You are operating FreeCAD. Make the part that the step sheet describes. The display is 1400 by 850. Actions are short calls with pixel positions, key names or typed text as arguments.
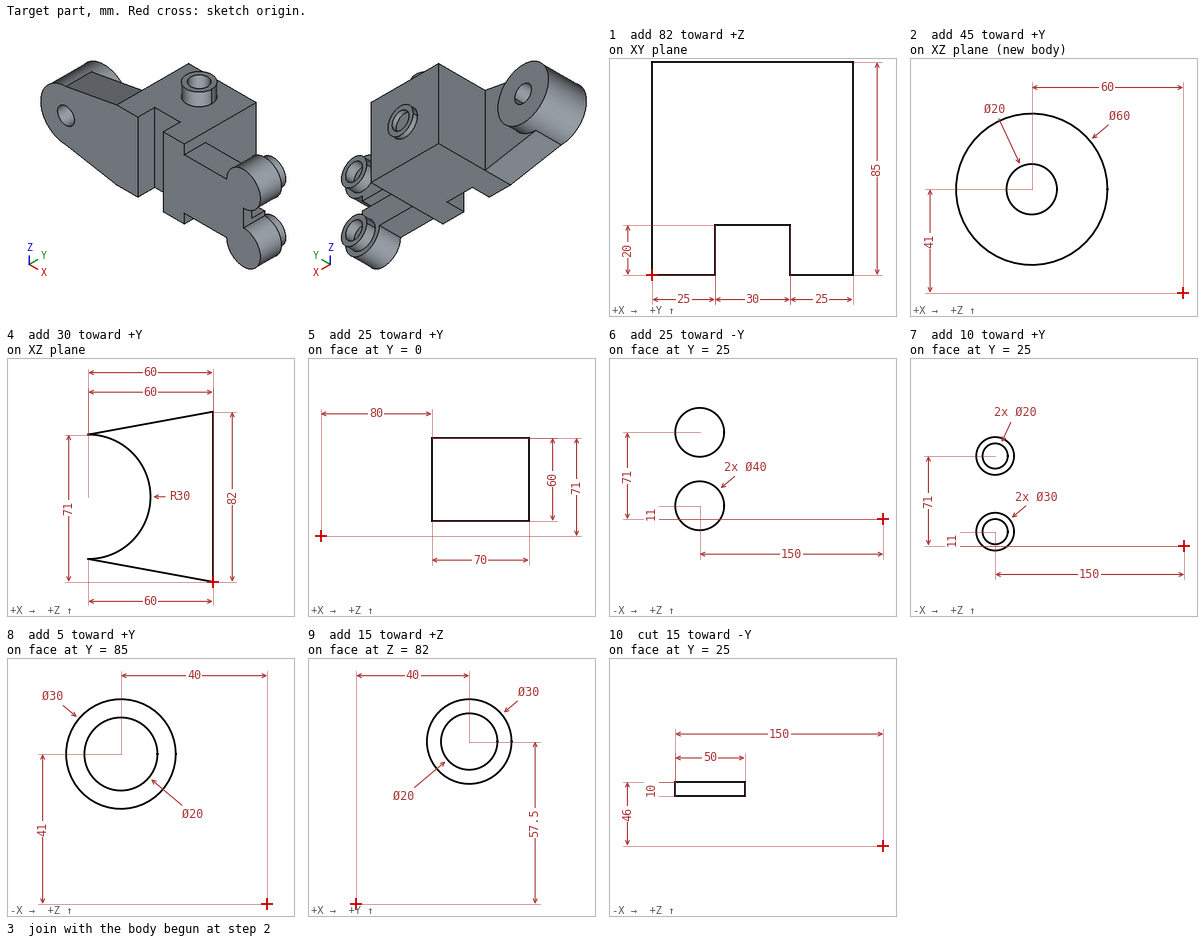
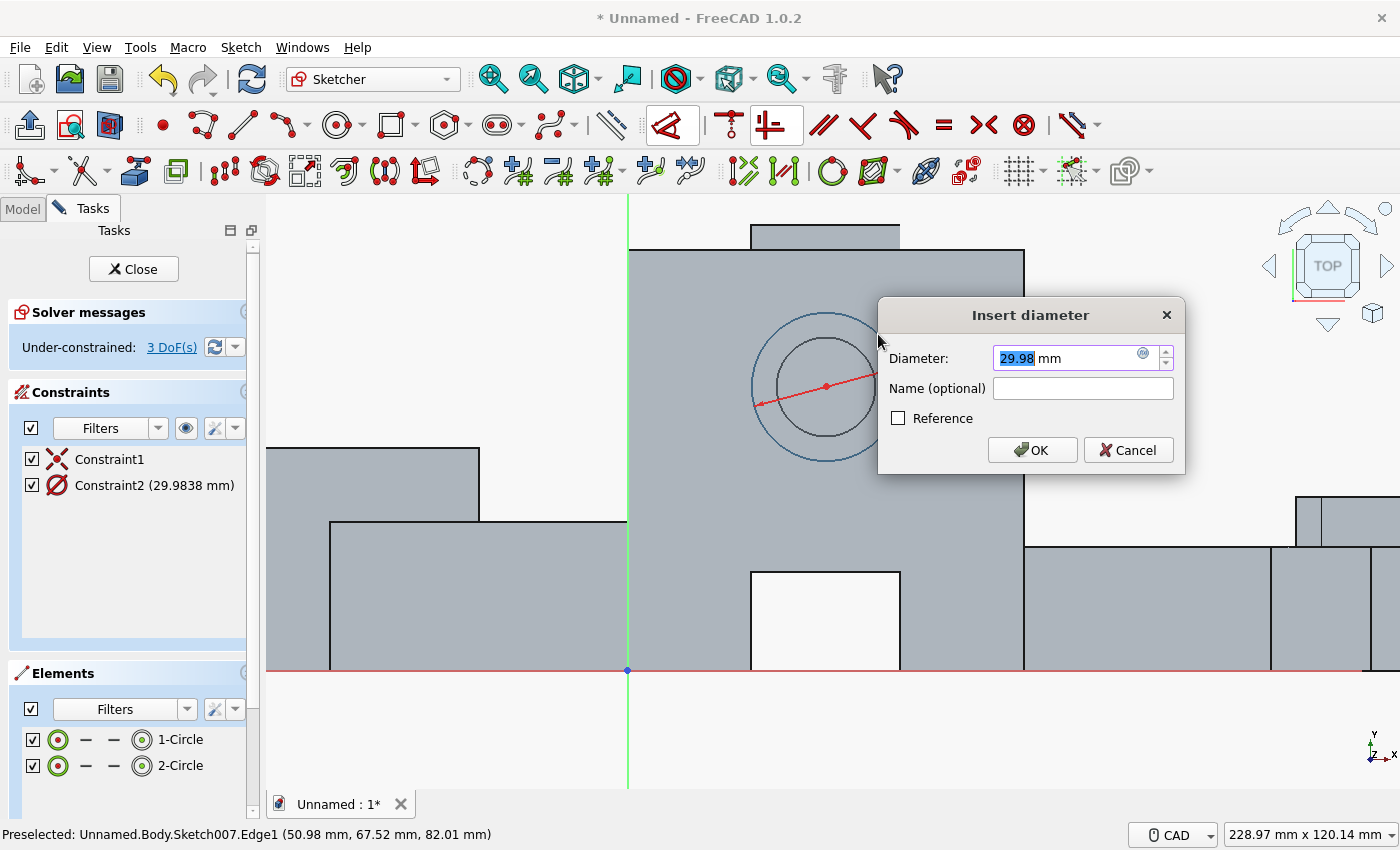
text(30)
key(Return)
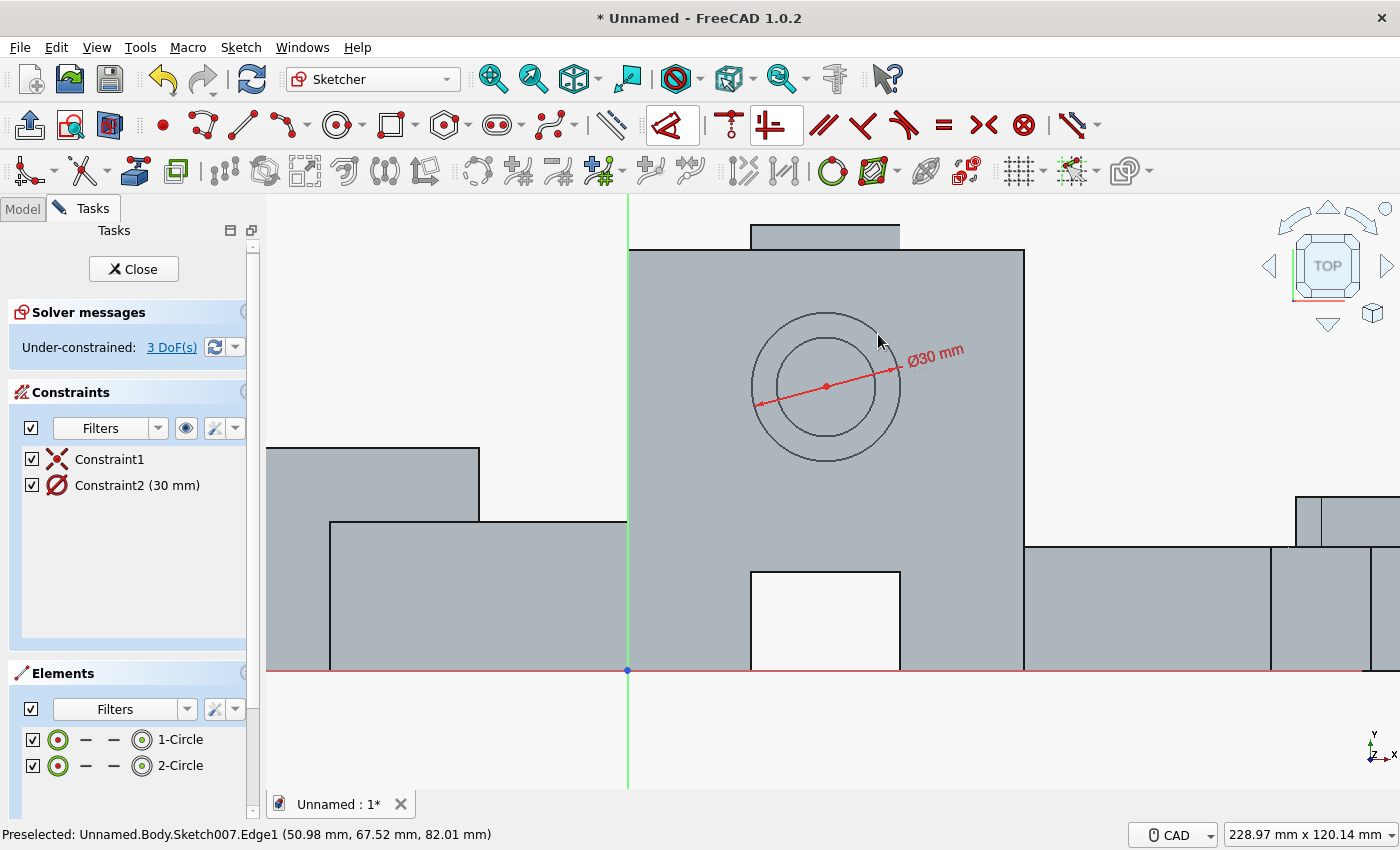
click(861, 352)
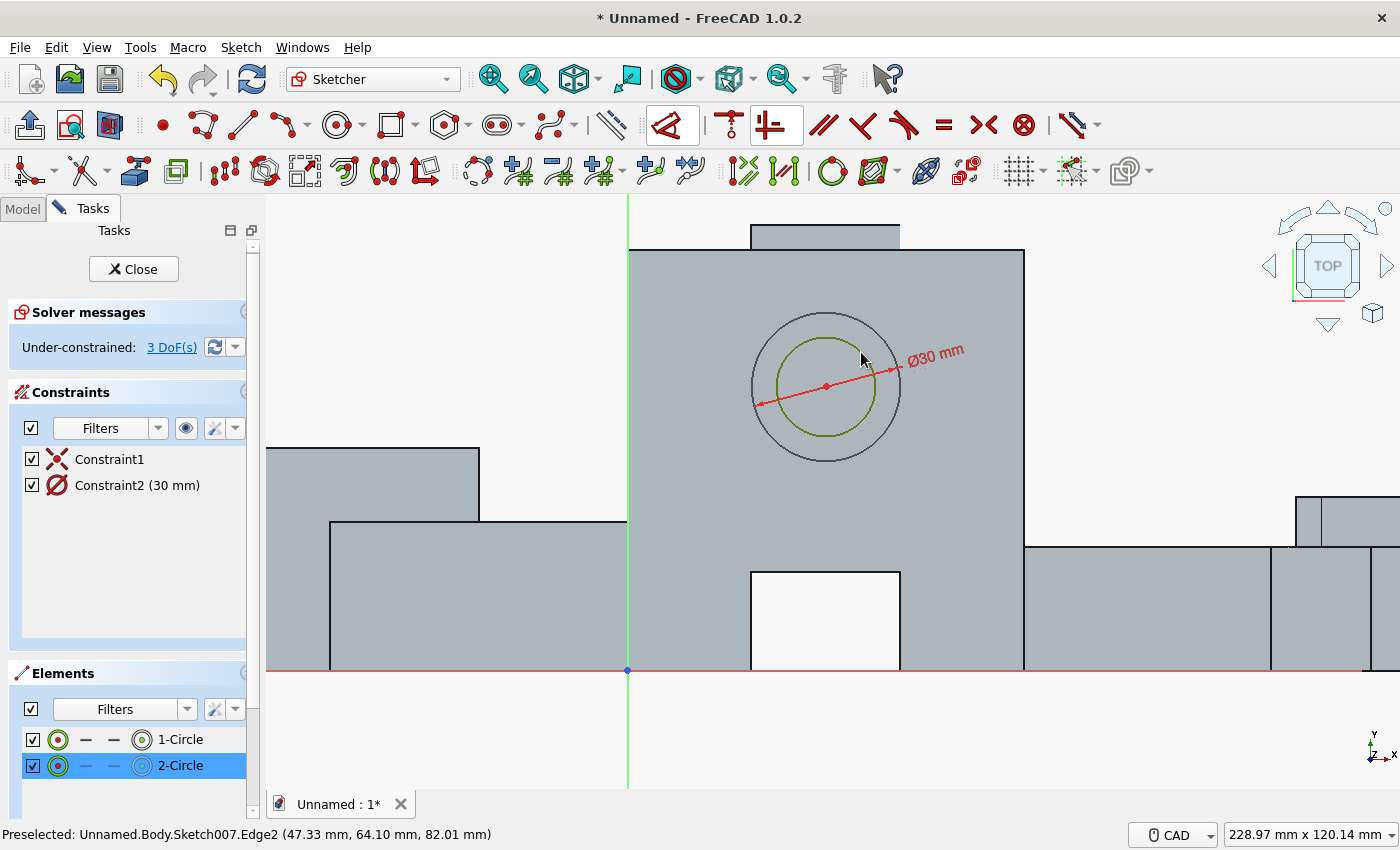
key(k)
key(o)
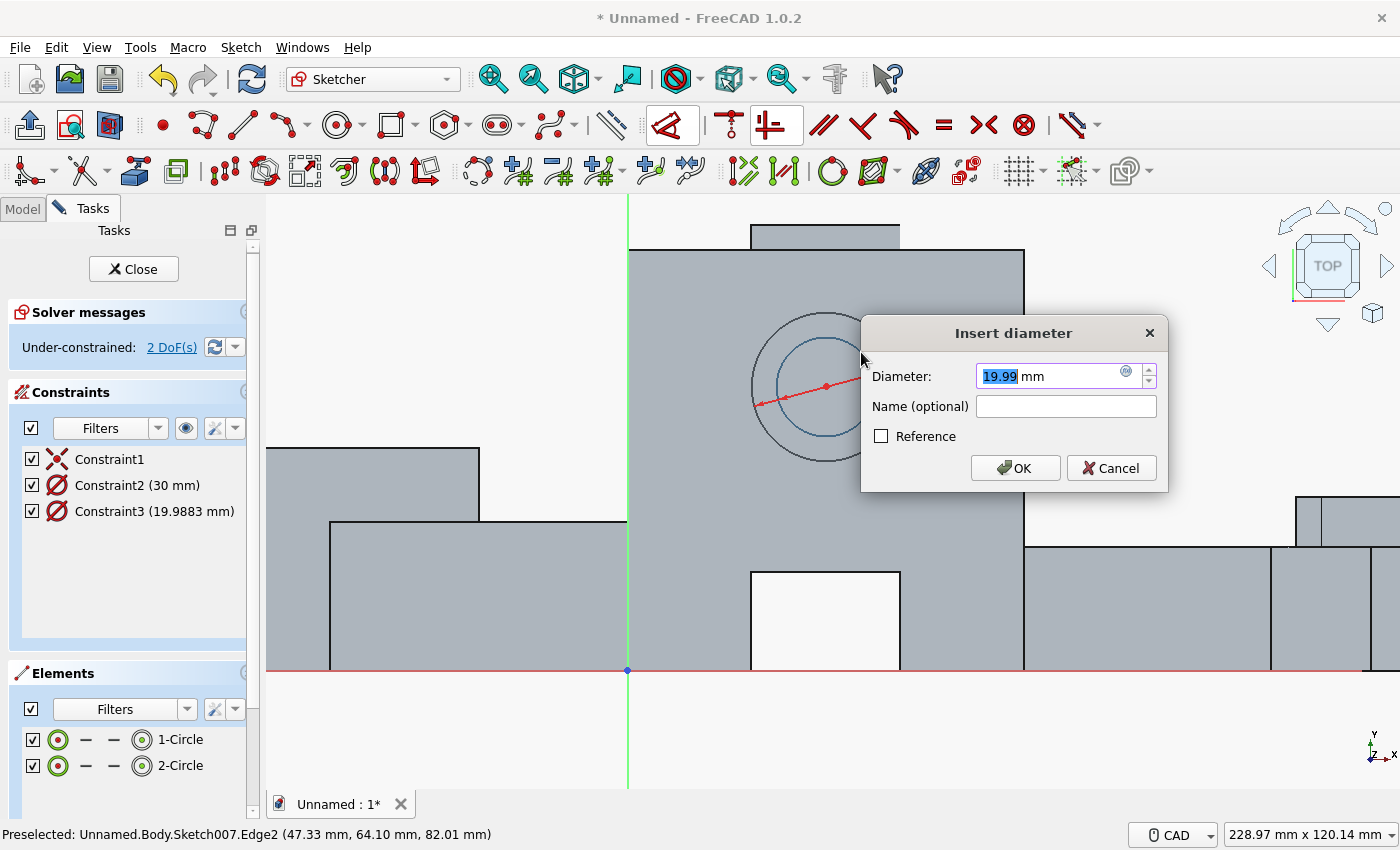
text(20)
key(Return)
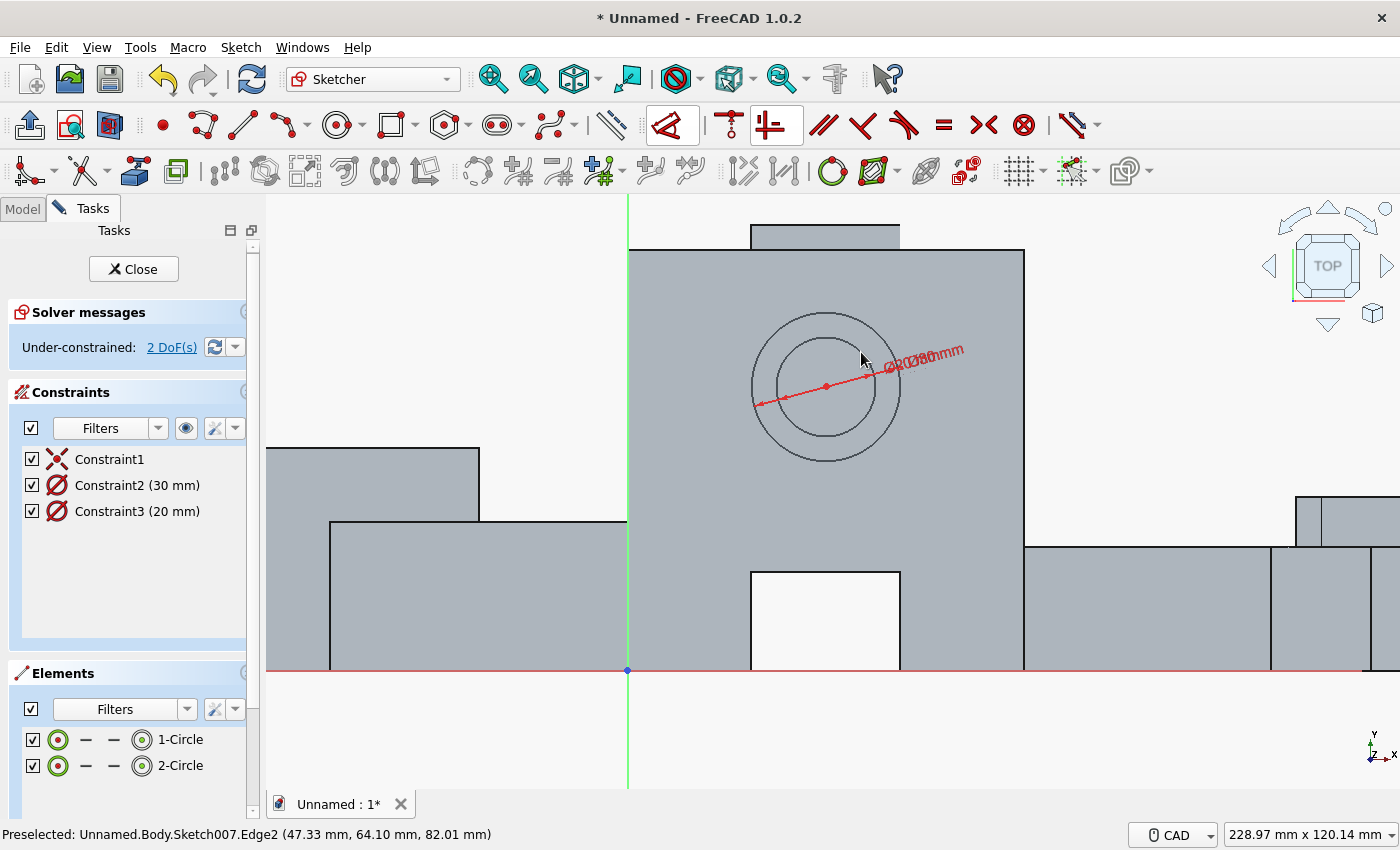
click(826, 387)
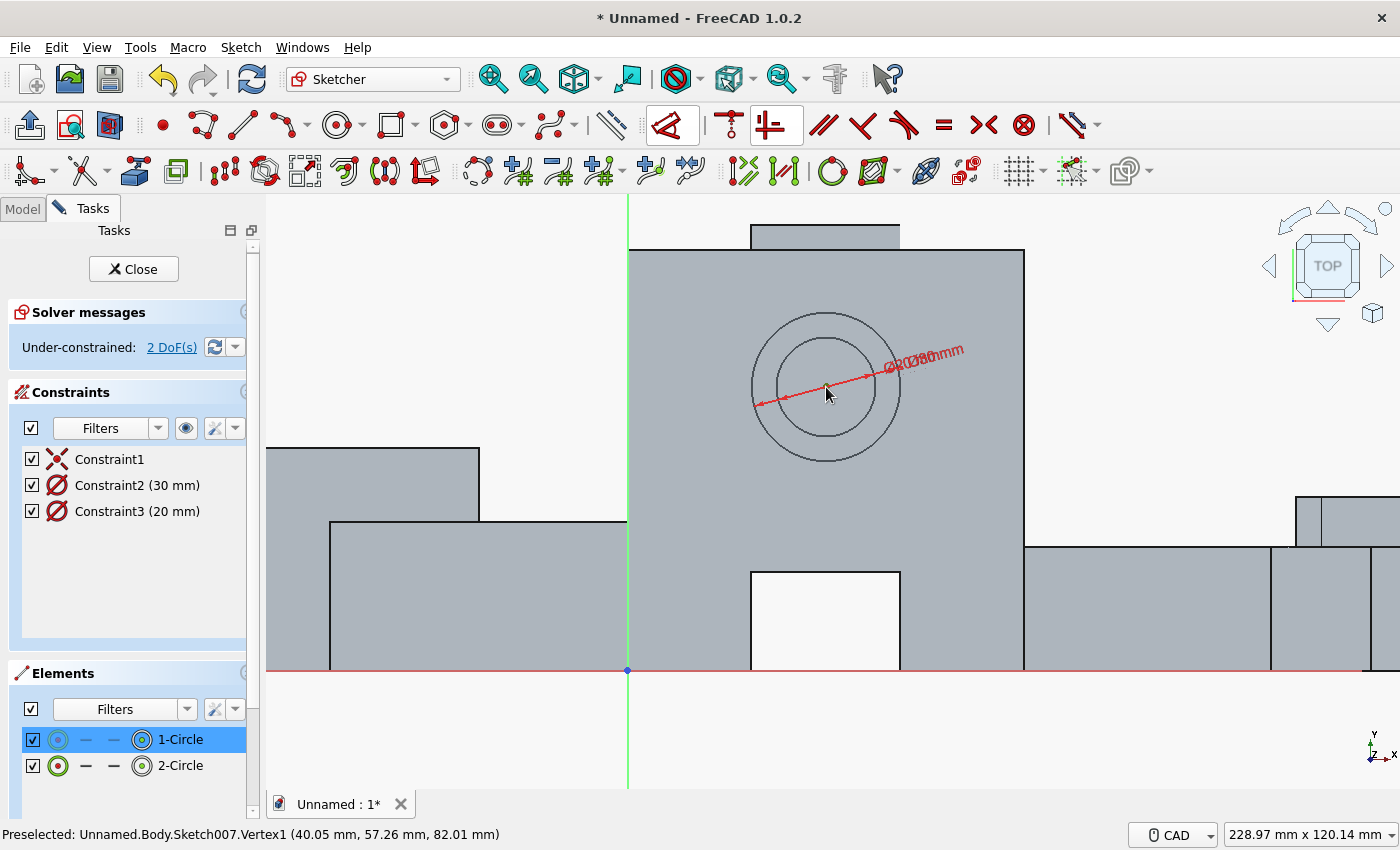
key(l)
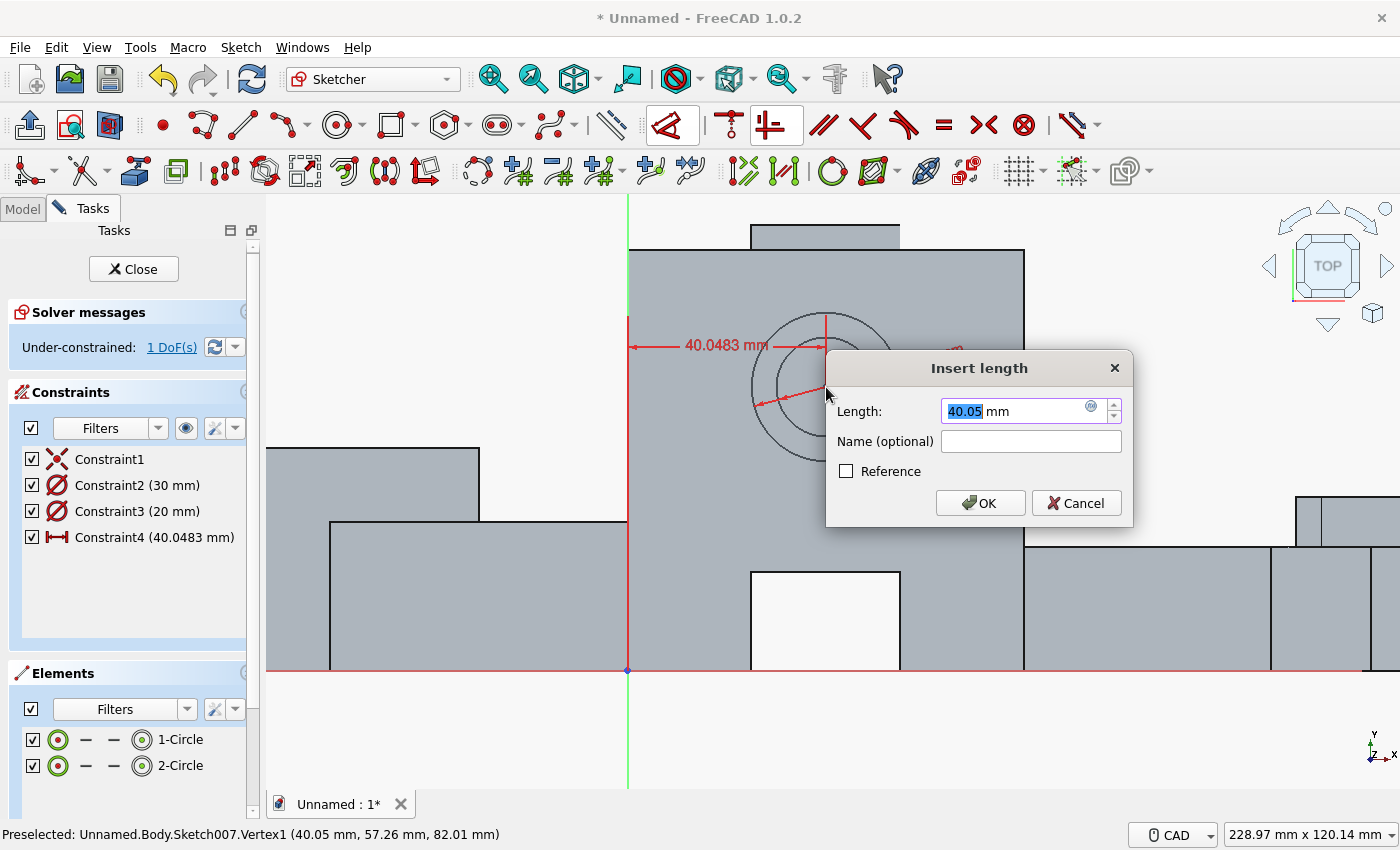
text(40)
key(Return)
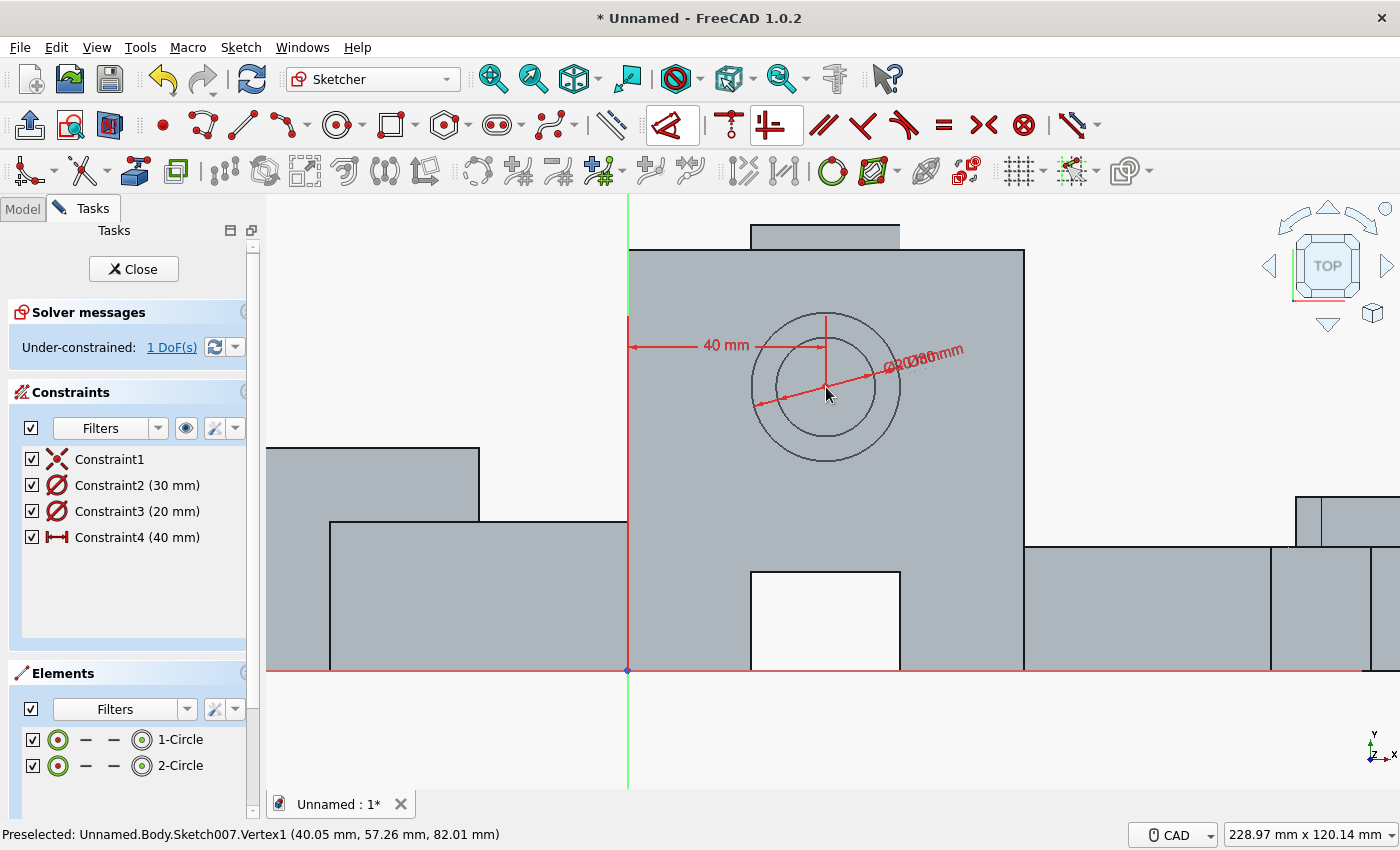
click(826, 387)